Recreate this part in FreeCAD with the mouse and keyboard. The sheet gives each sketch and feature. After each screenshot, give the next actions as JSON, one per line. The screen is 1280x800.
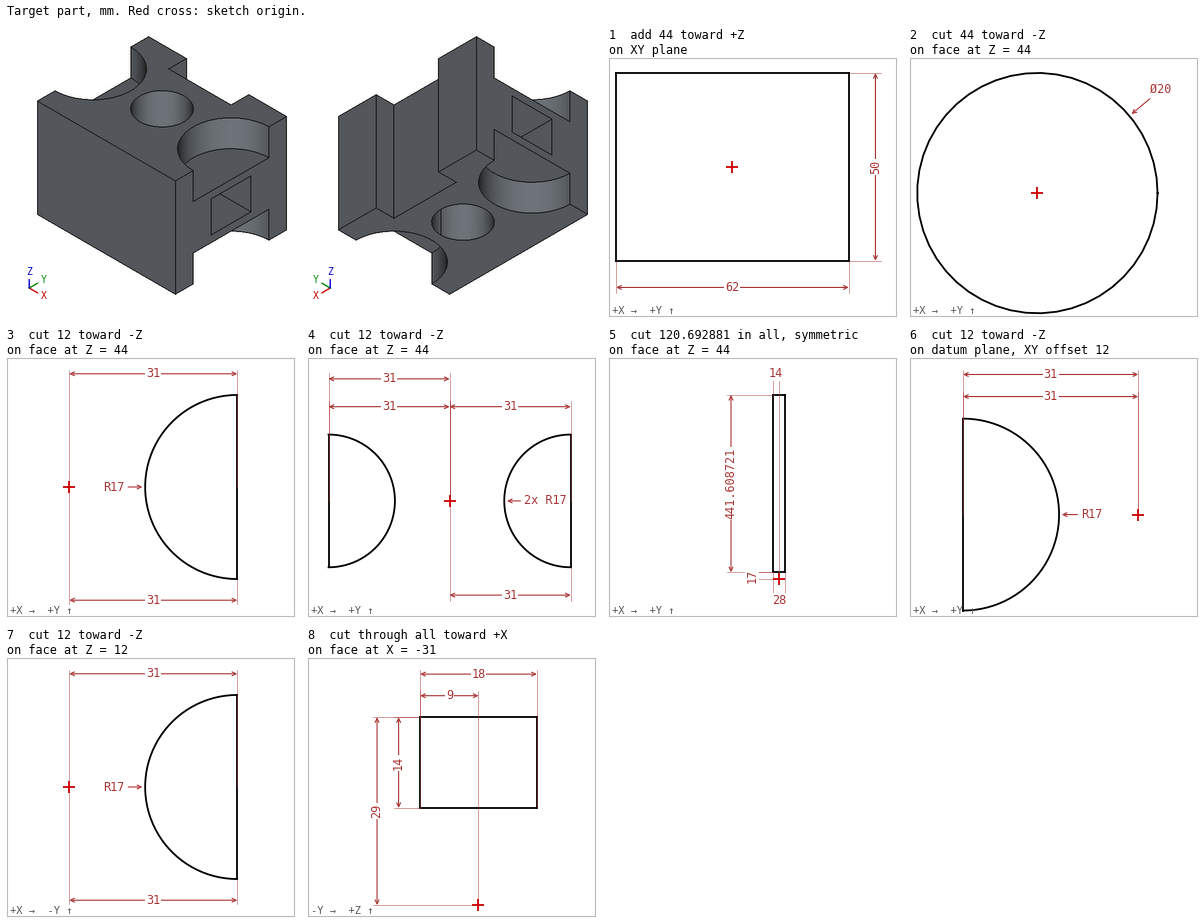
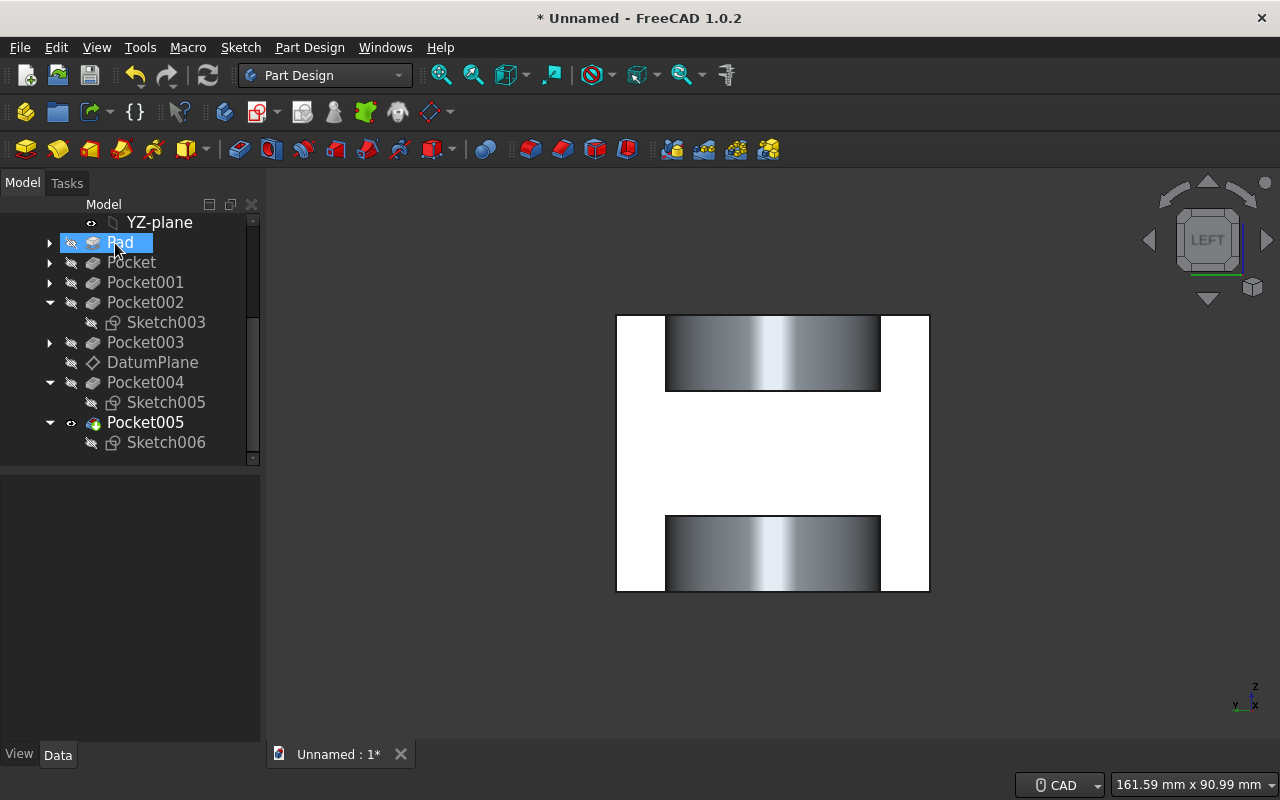
{"action": "left_click", "coordinate": [683, 452]}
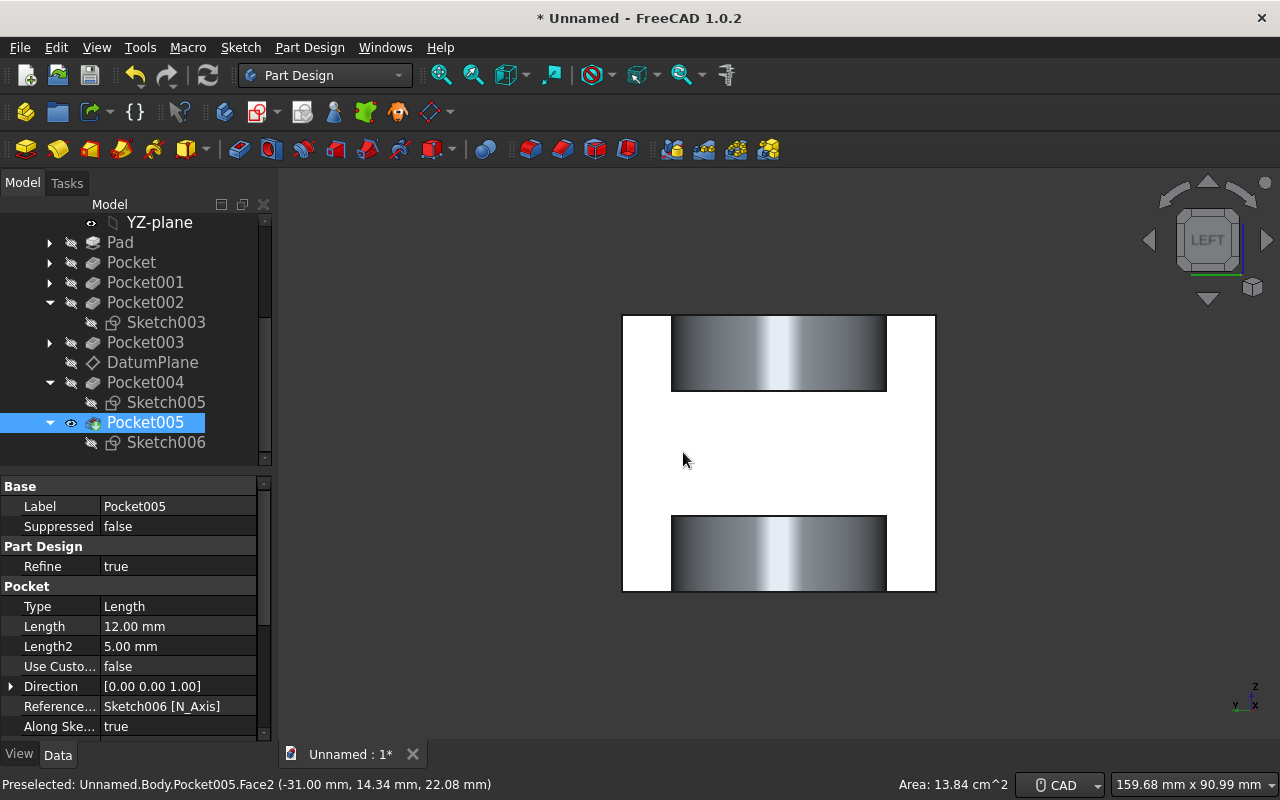
{"action": "left_click", "coordinate": [258, 112]}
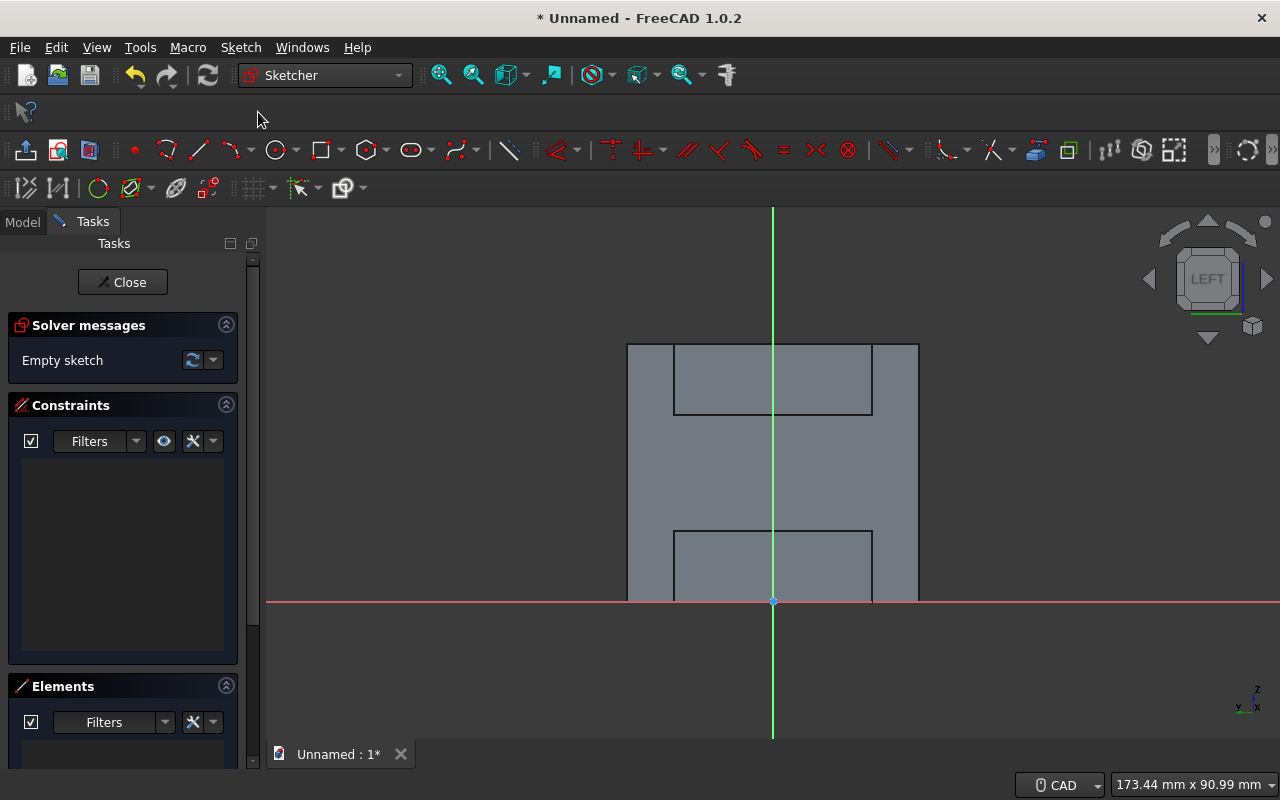
{"action": "scroll", "coordinate": [856, 570], "scroll_direction": "up", "scroll_amount": 3}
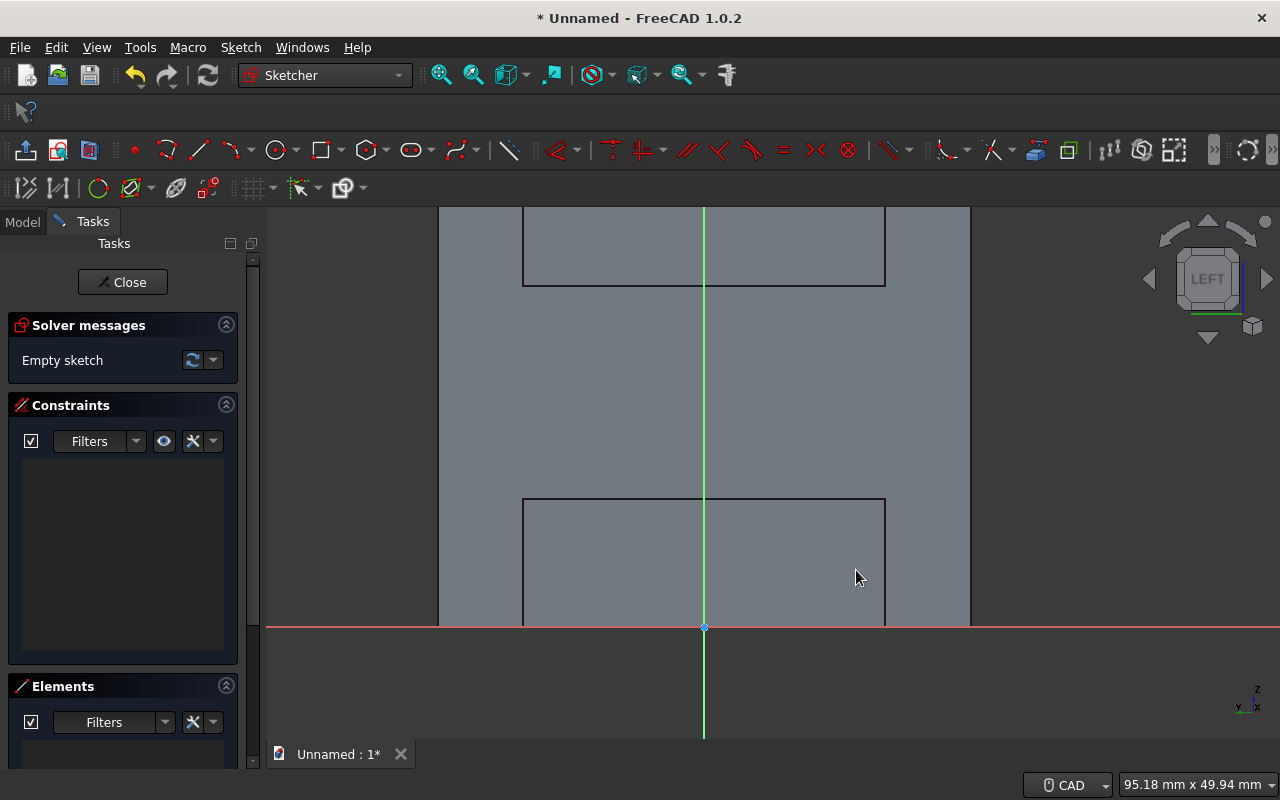
{"action": "key", "text": "g r"}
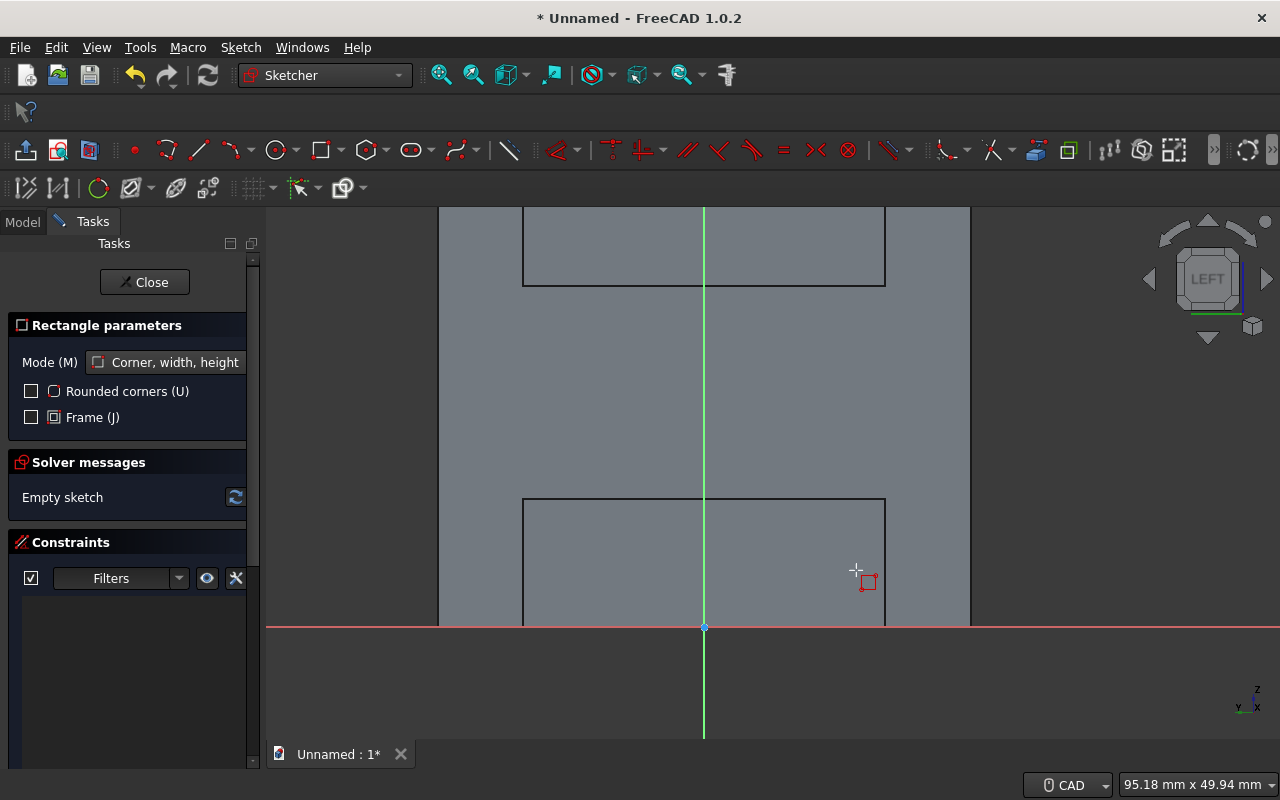
{"action": "left_click", "coordinate": [608, 318]}
{"action": "left_click", "coordinate": [800, 467]}
{"action": "key", "text": "Escape"}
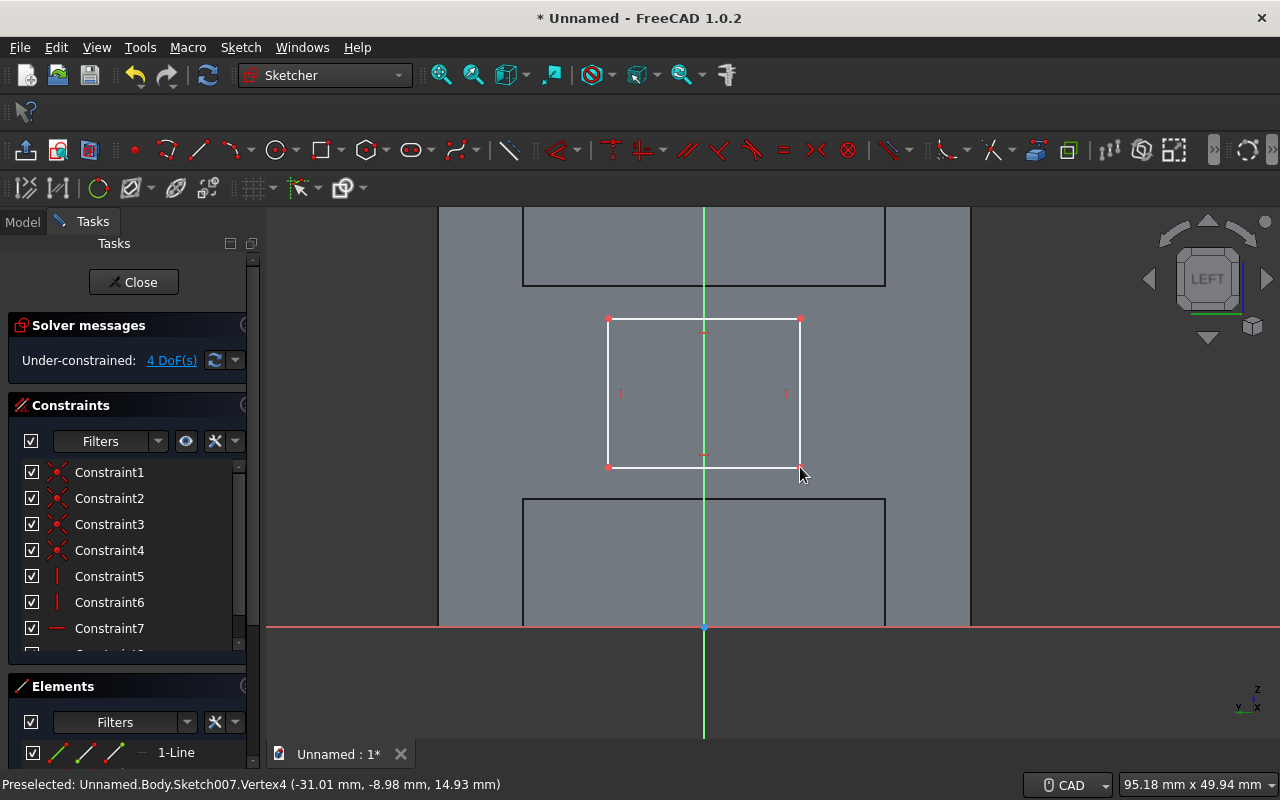
{"action": "key", "text": "d"}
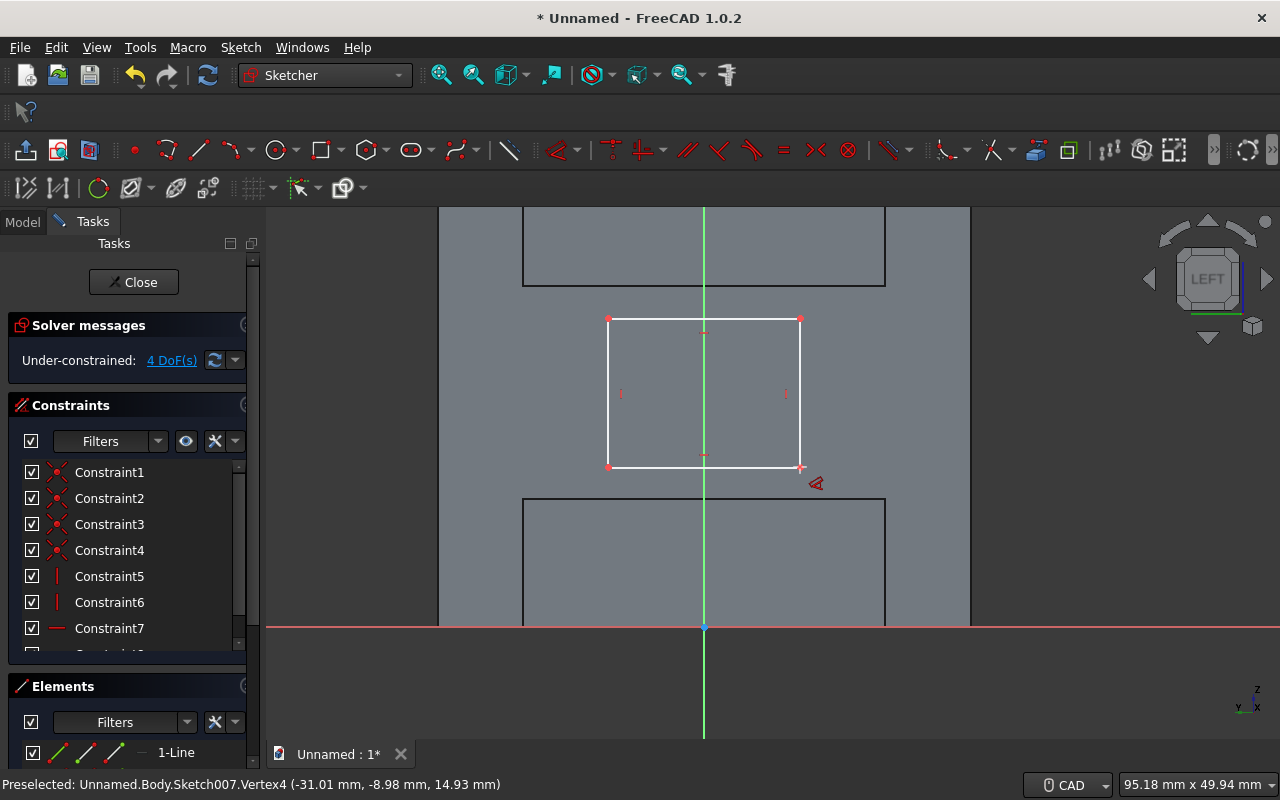
{"action": "left_click", "coordinate": [608, 364]}
{"action": "left_click", "coordinate": [574, 393]}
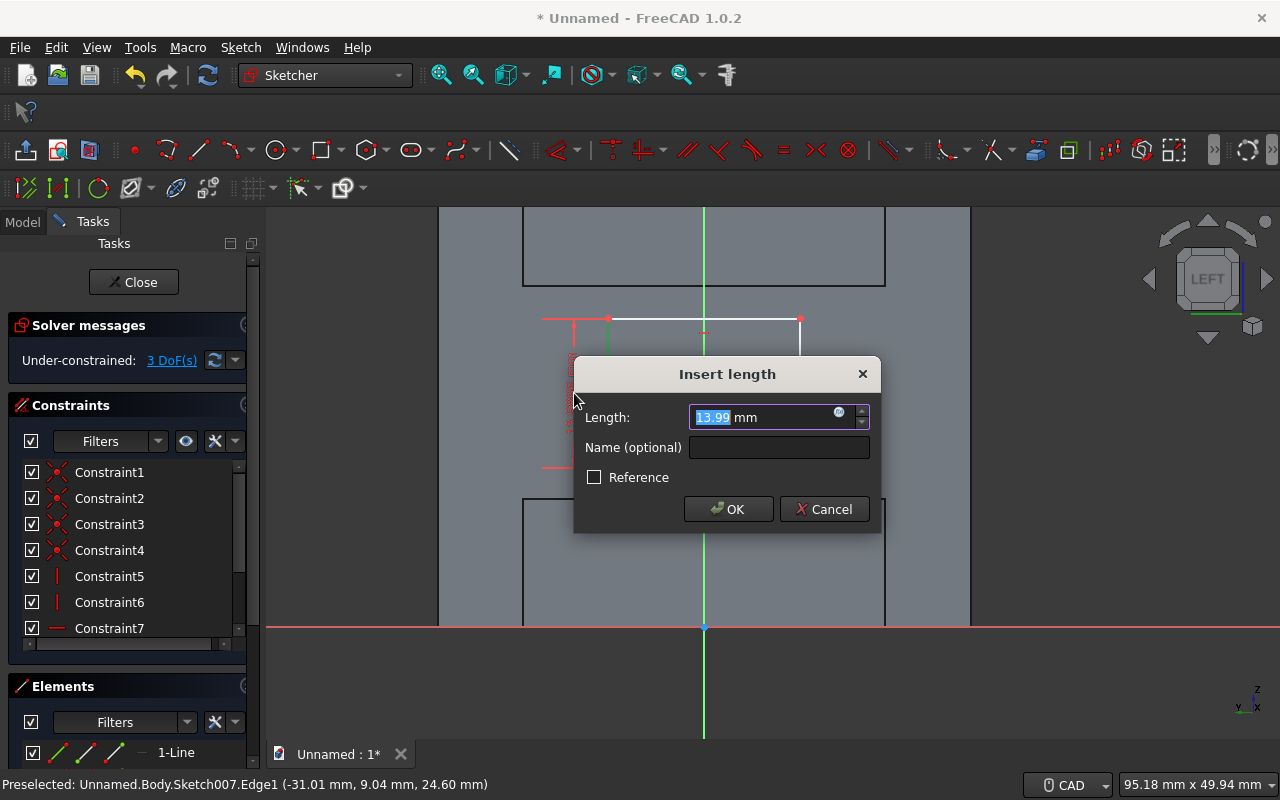
{"action": "type", "text": "14"}
{"action": "key", "text": "Return"}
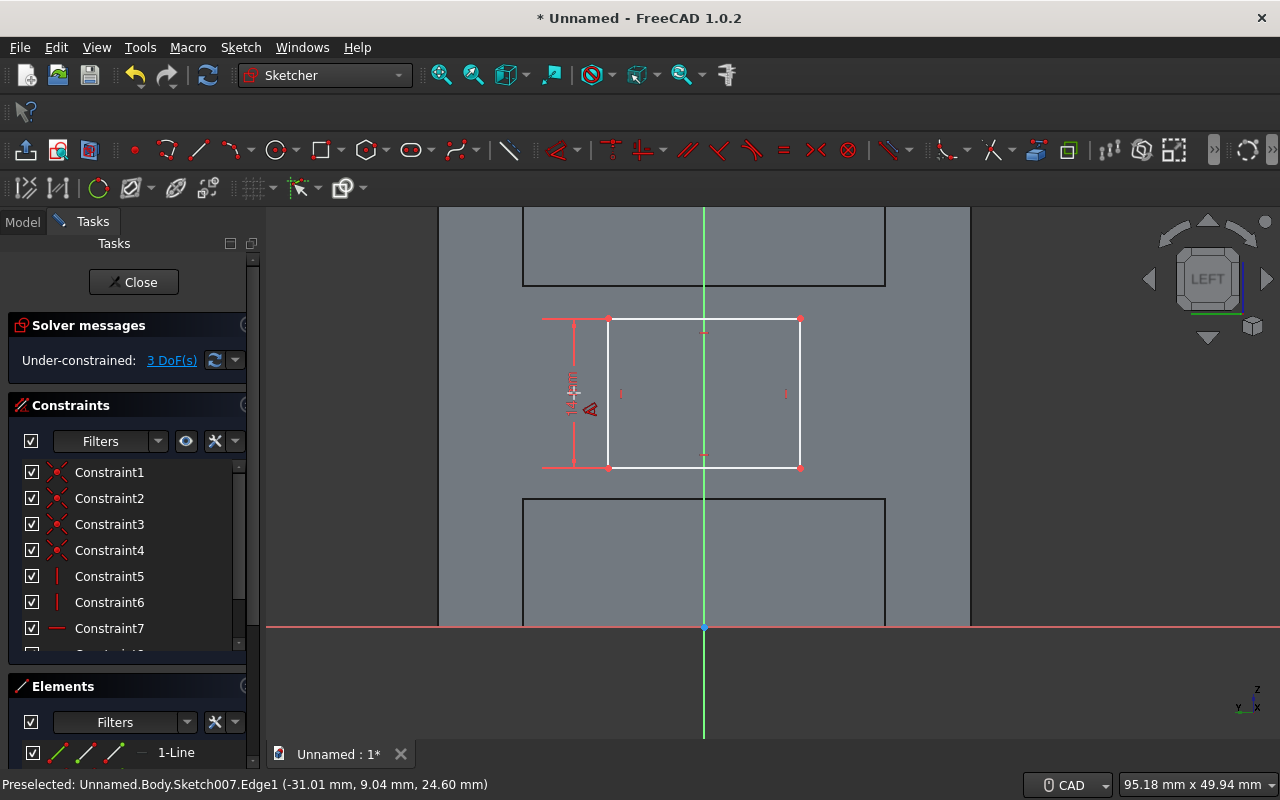
{"action": "left_click", "coordinate": [666, 468]}
{"action": "left_click", "coordinate": [660, 434]}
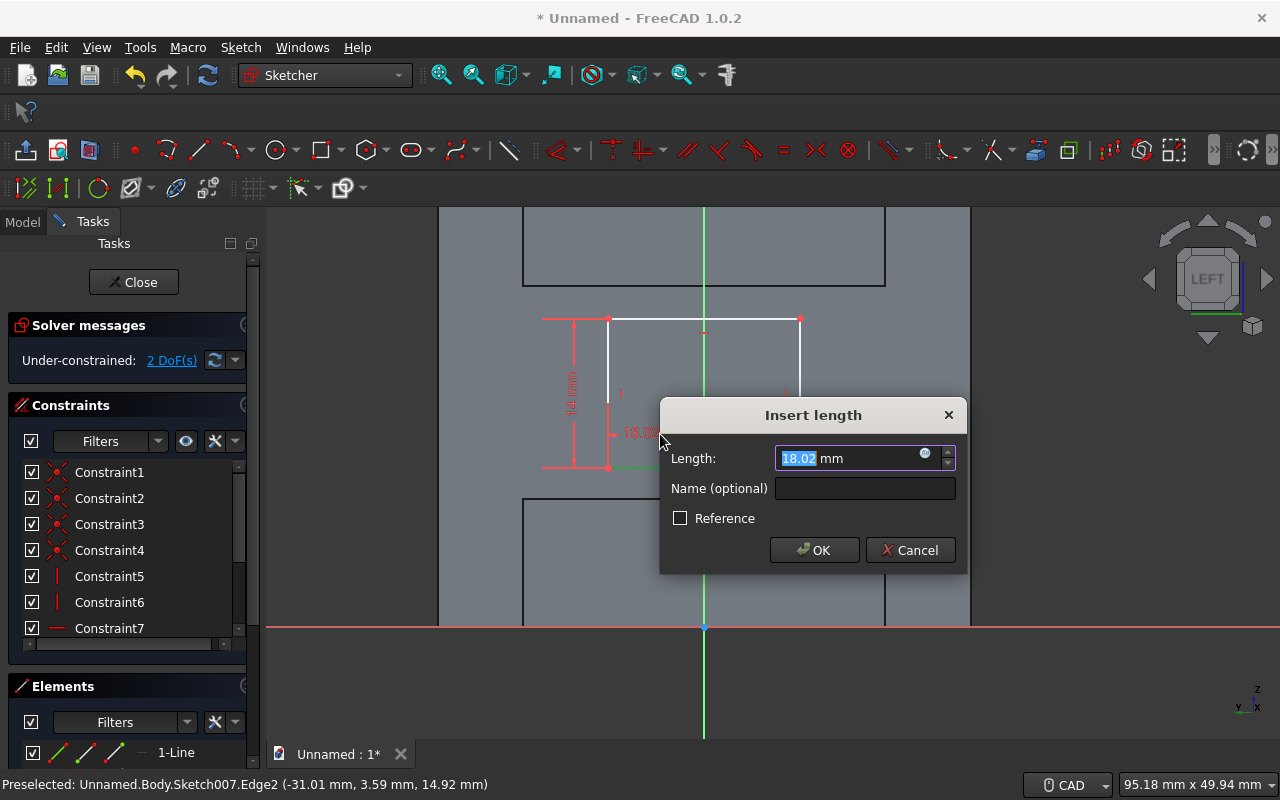
{"action": "type", "text": "18"}
{"action": "key", "text": "Return"}